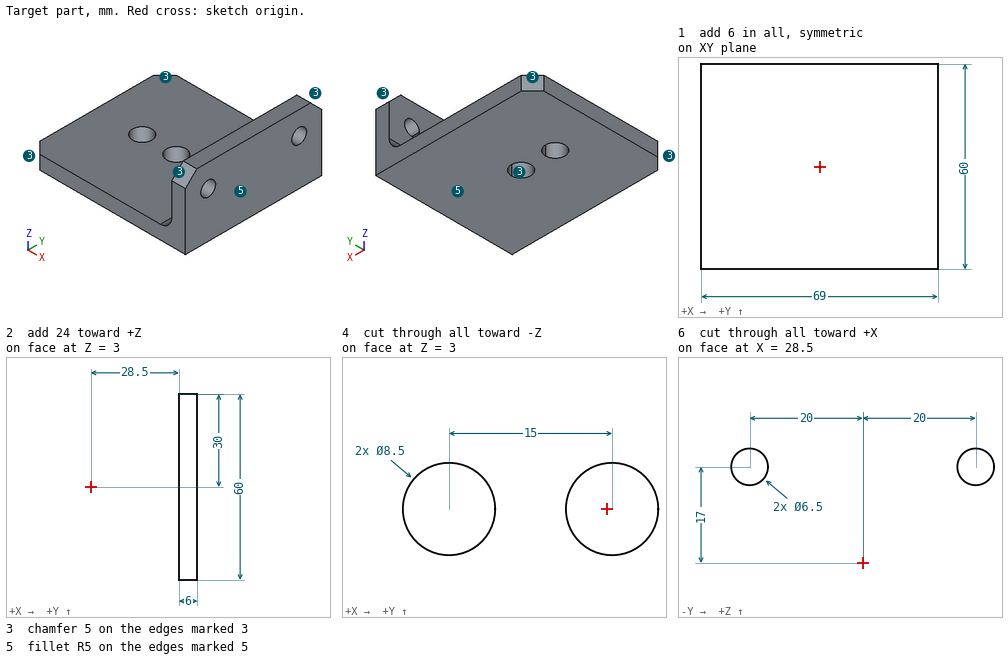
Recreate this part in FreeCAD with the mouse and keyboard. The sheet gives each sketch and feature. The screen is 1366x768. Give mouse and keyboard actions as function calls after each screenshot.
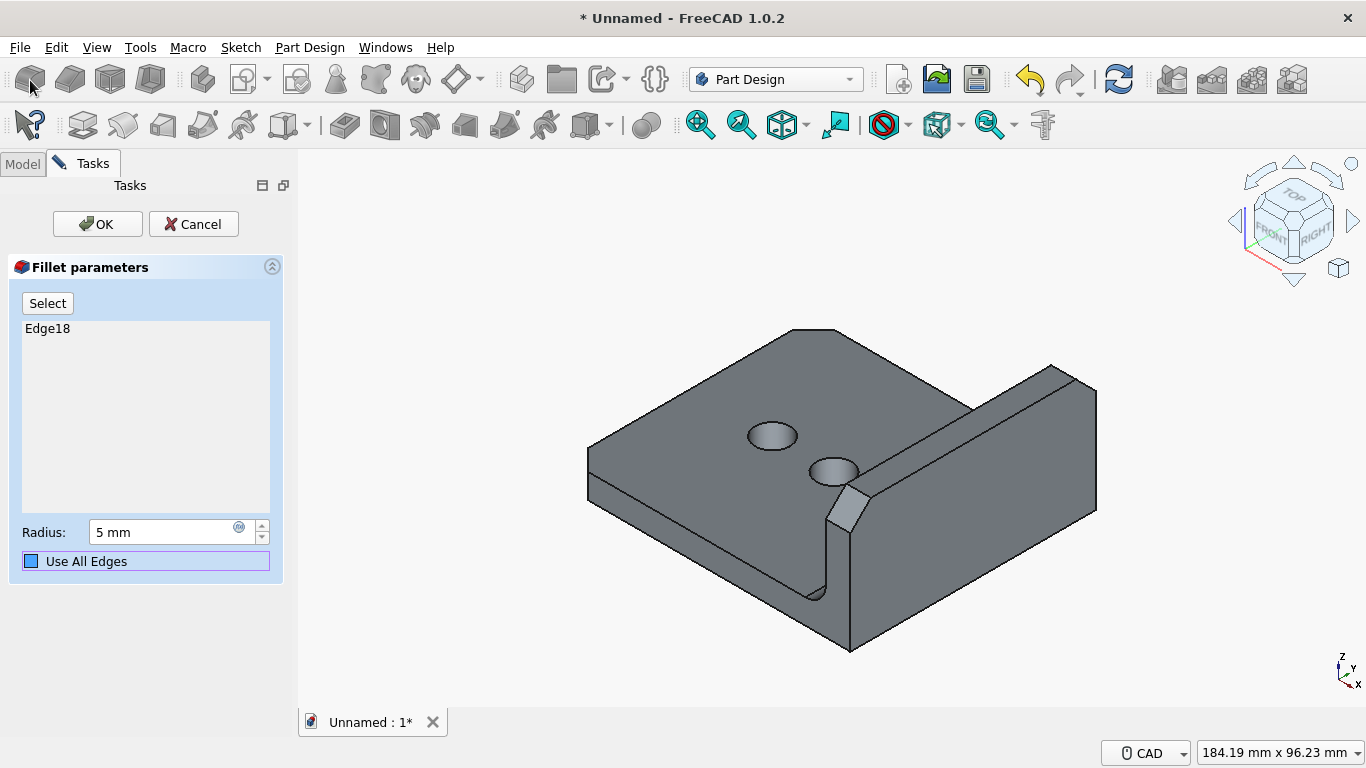
click(98, 224)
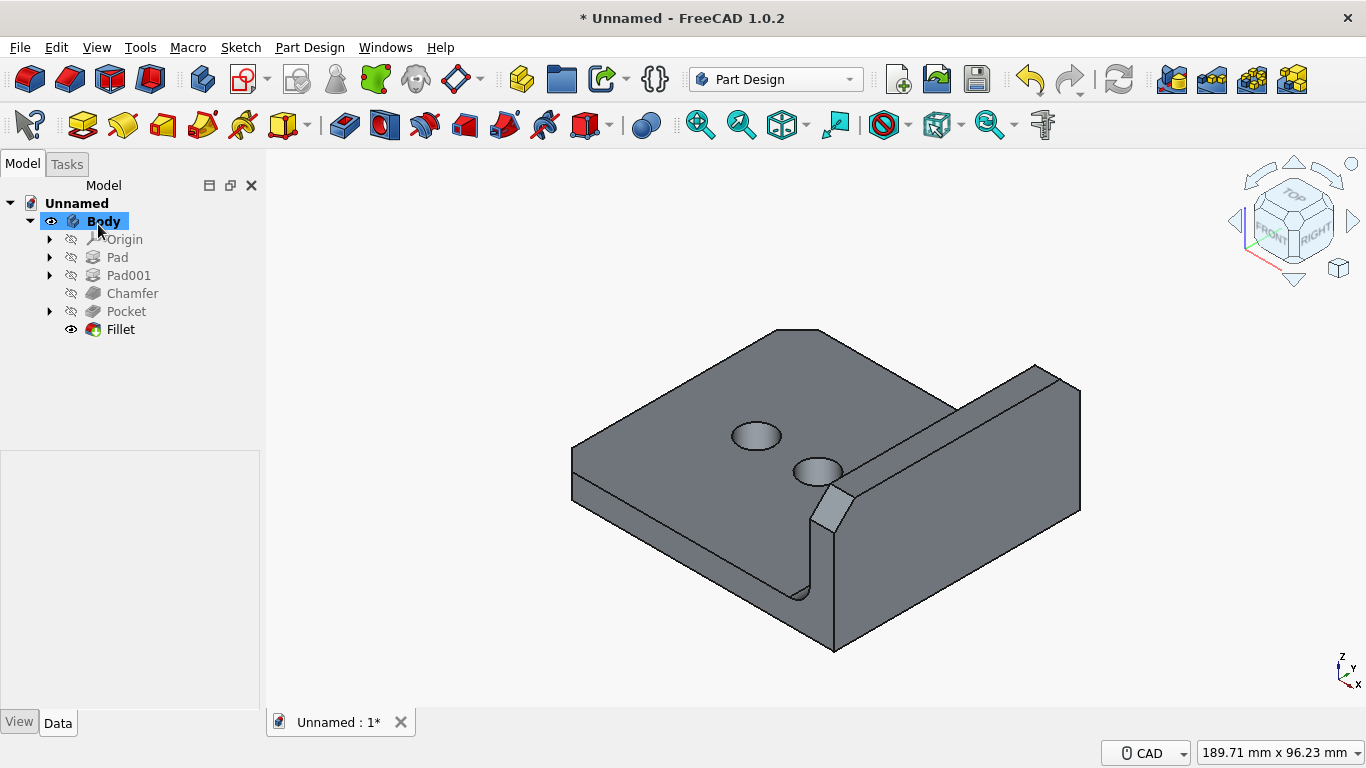
key(6)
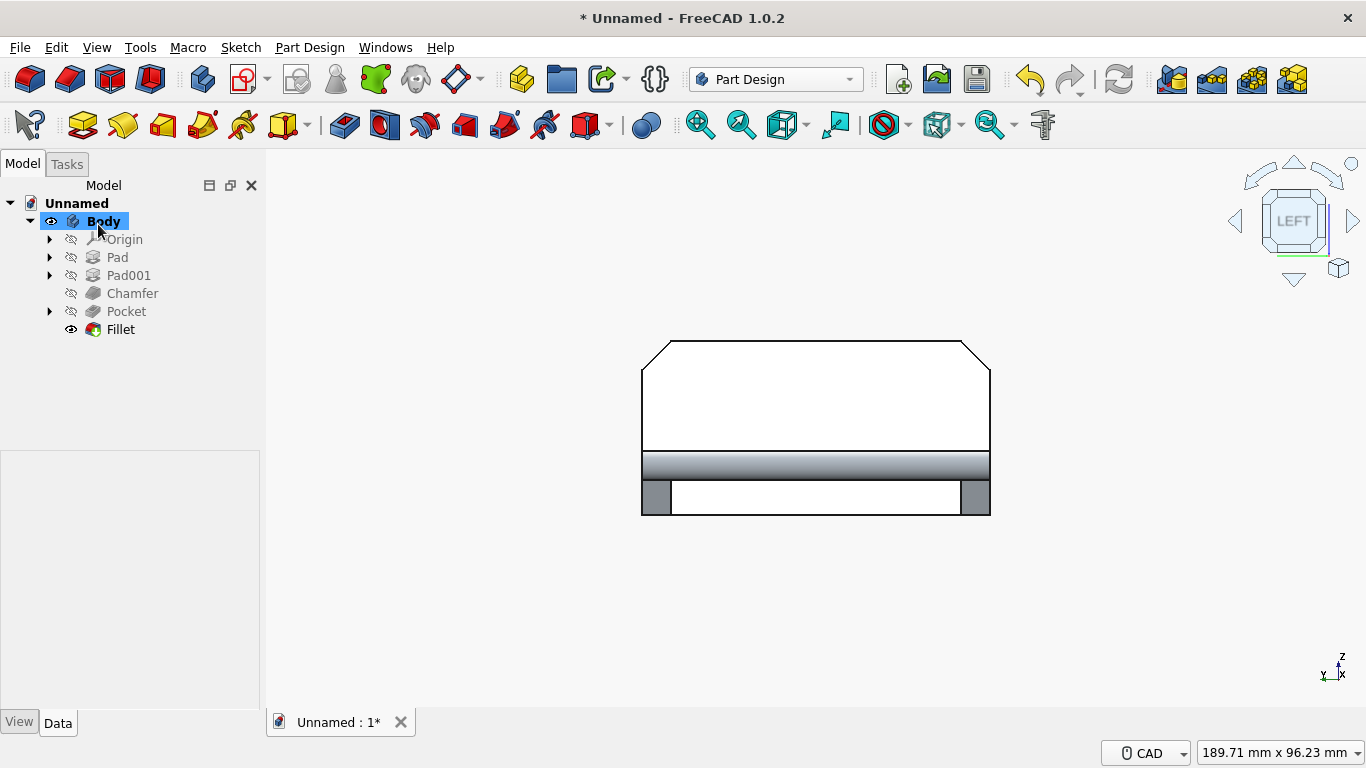
click(702, 126)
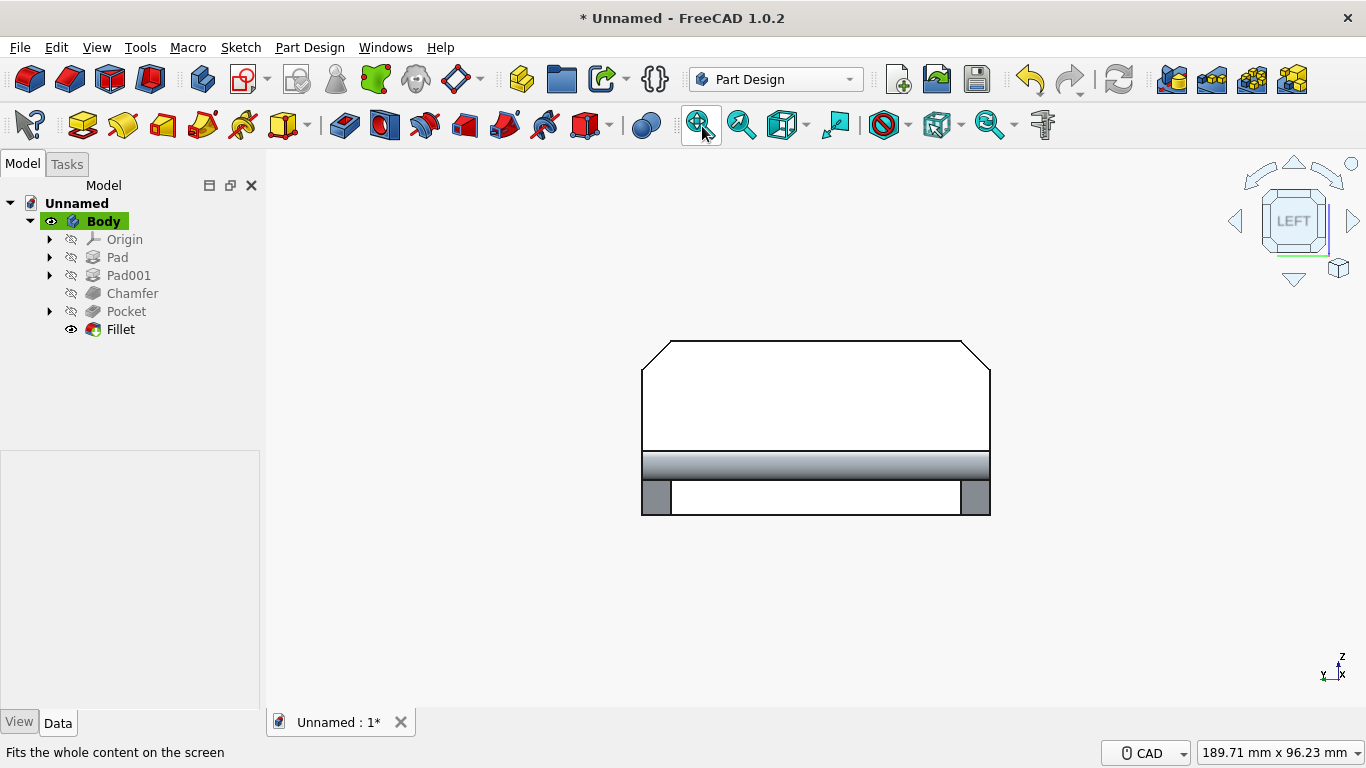
click(717, 395)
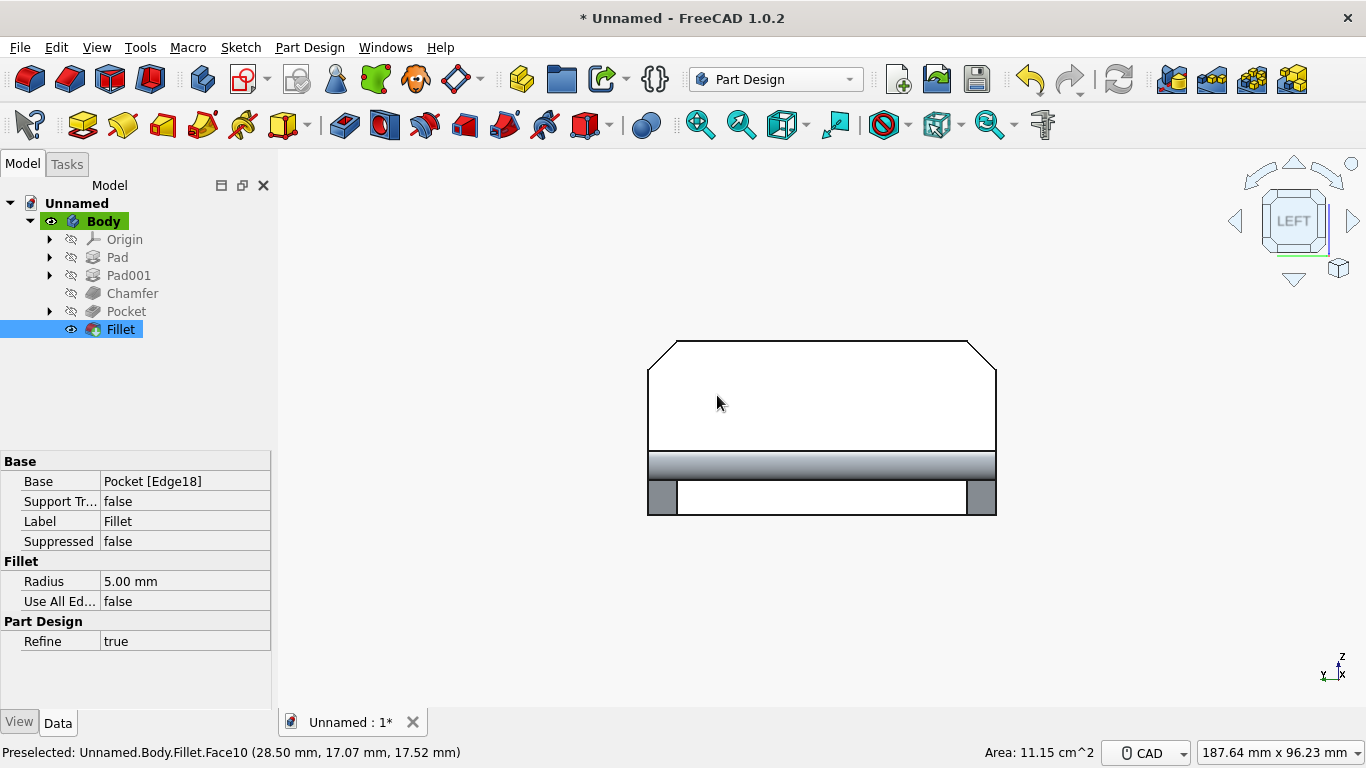
click(244, 80)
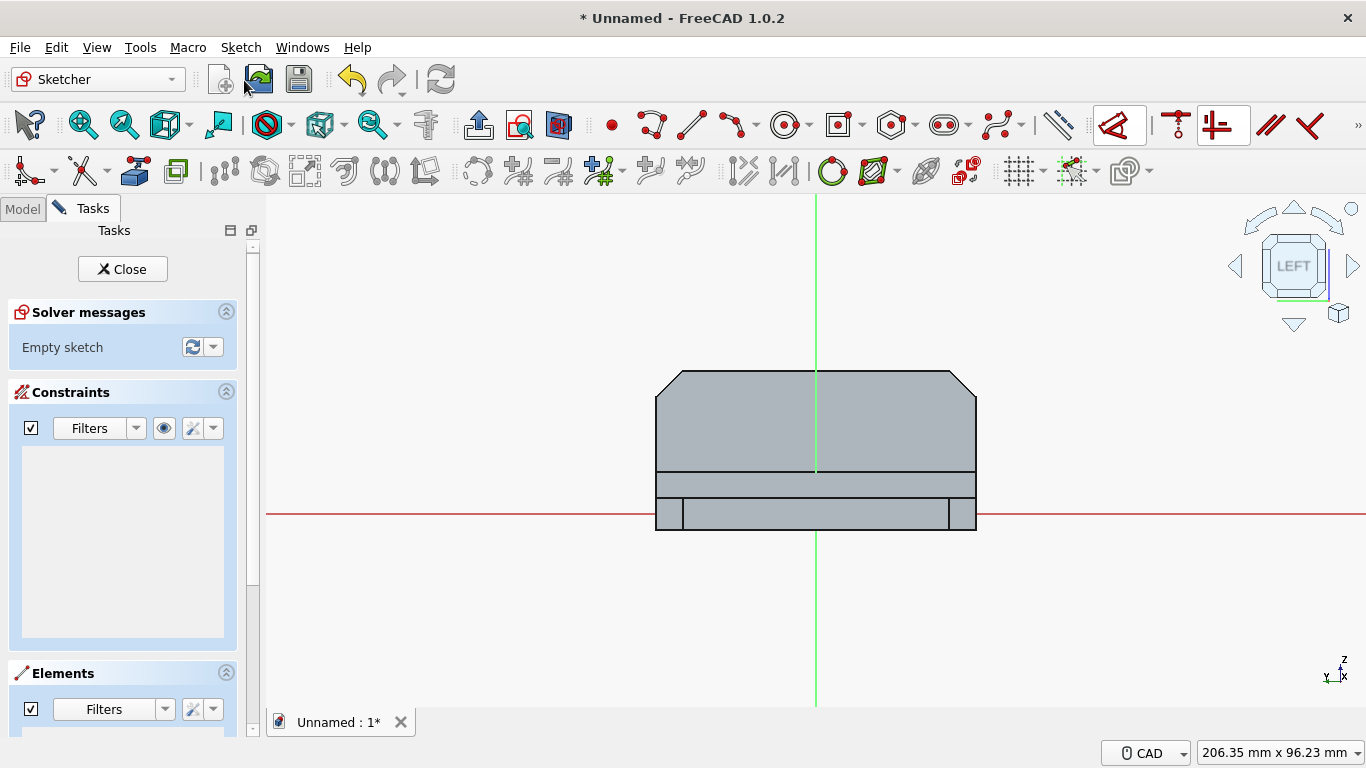
scroll(856, 466, up, 5)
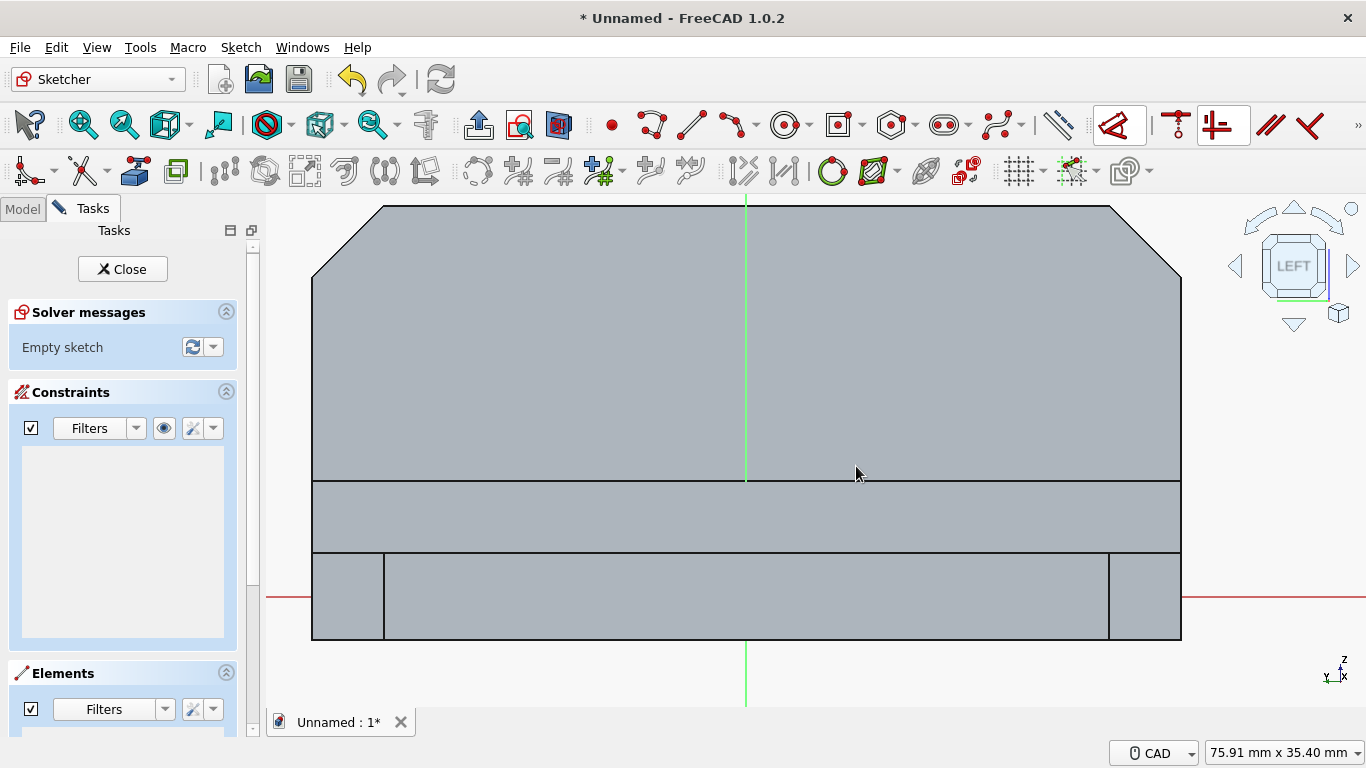
click(786, 126)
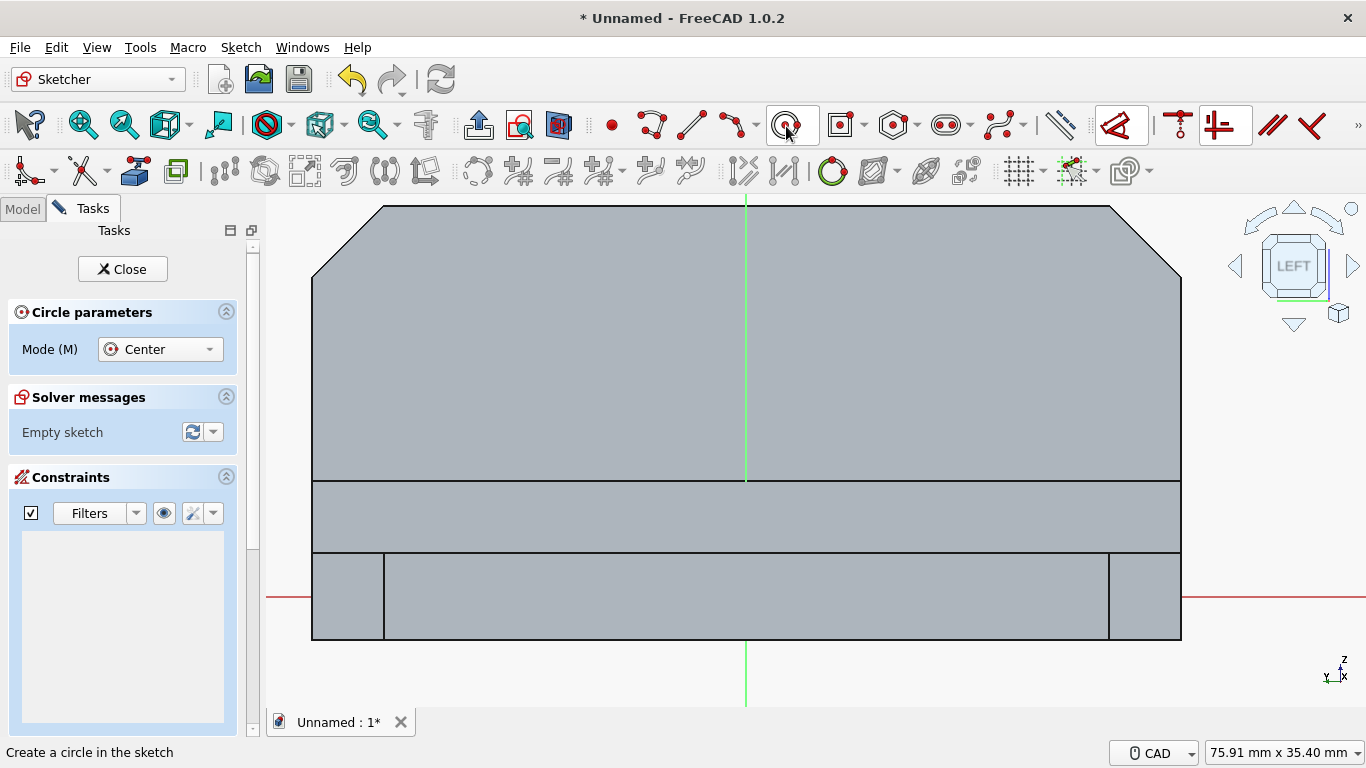
click(457, 351)
move(490, 317)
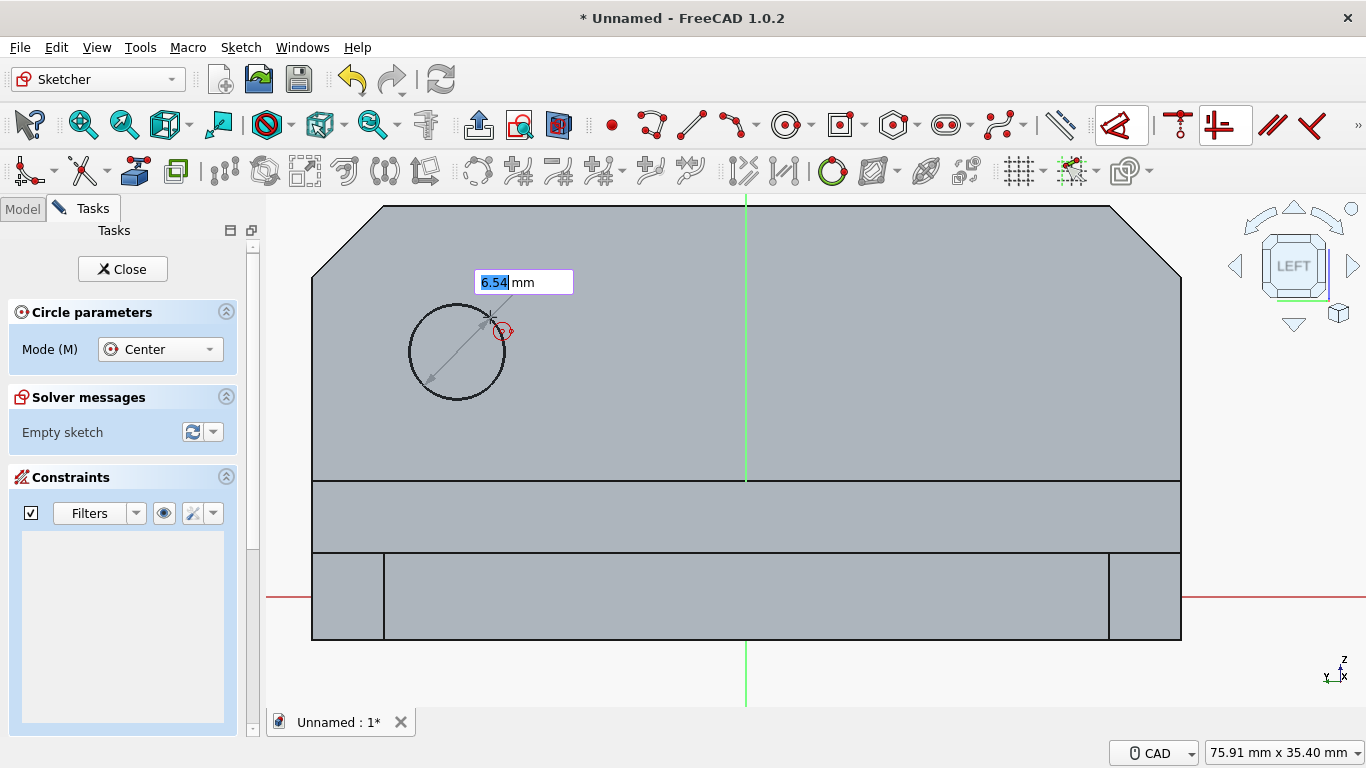
text(6.5)
key(Return)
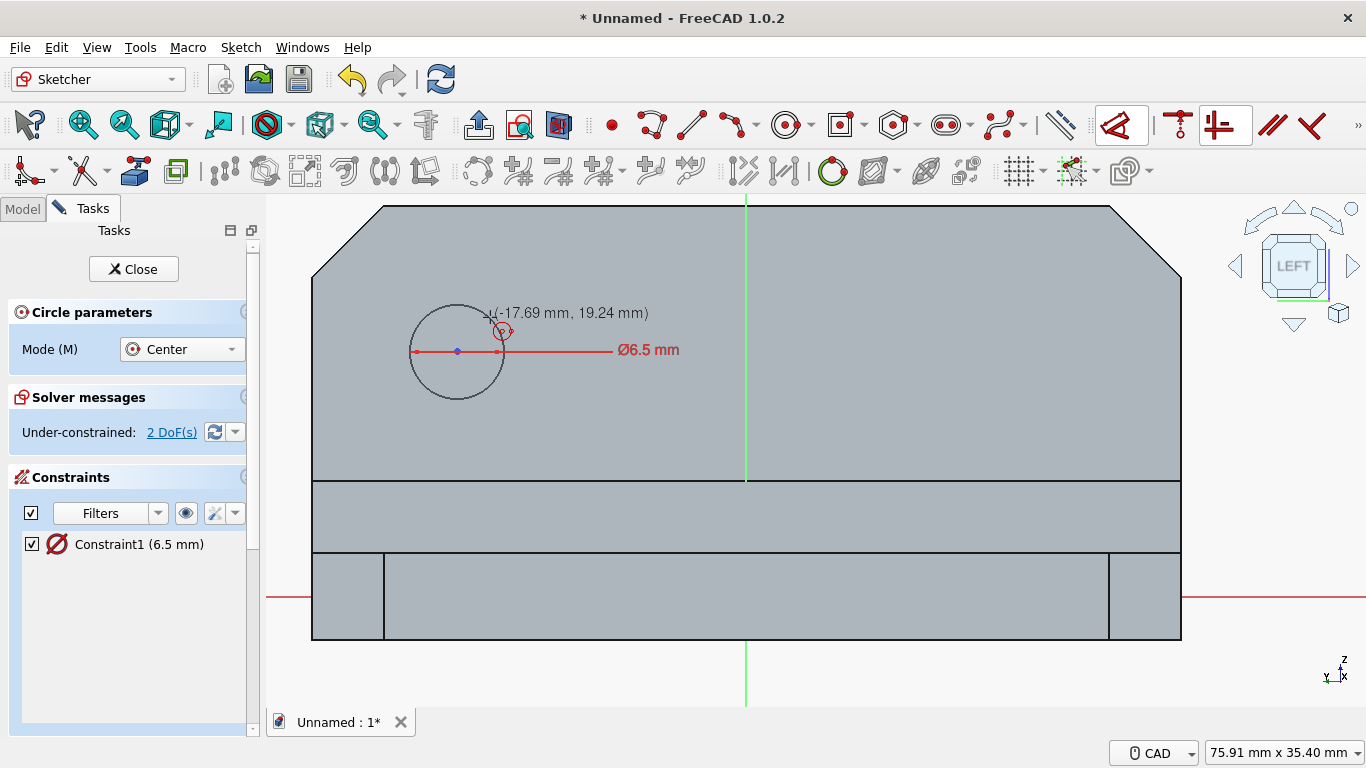
click(1036, 351)
move(1069, 317)